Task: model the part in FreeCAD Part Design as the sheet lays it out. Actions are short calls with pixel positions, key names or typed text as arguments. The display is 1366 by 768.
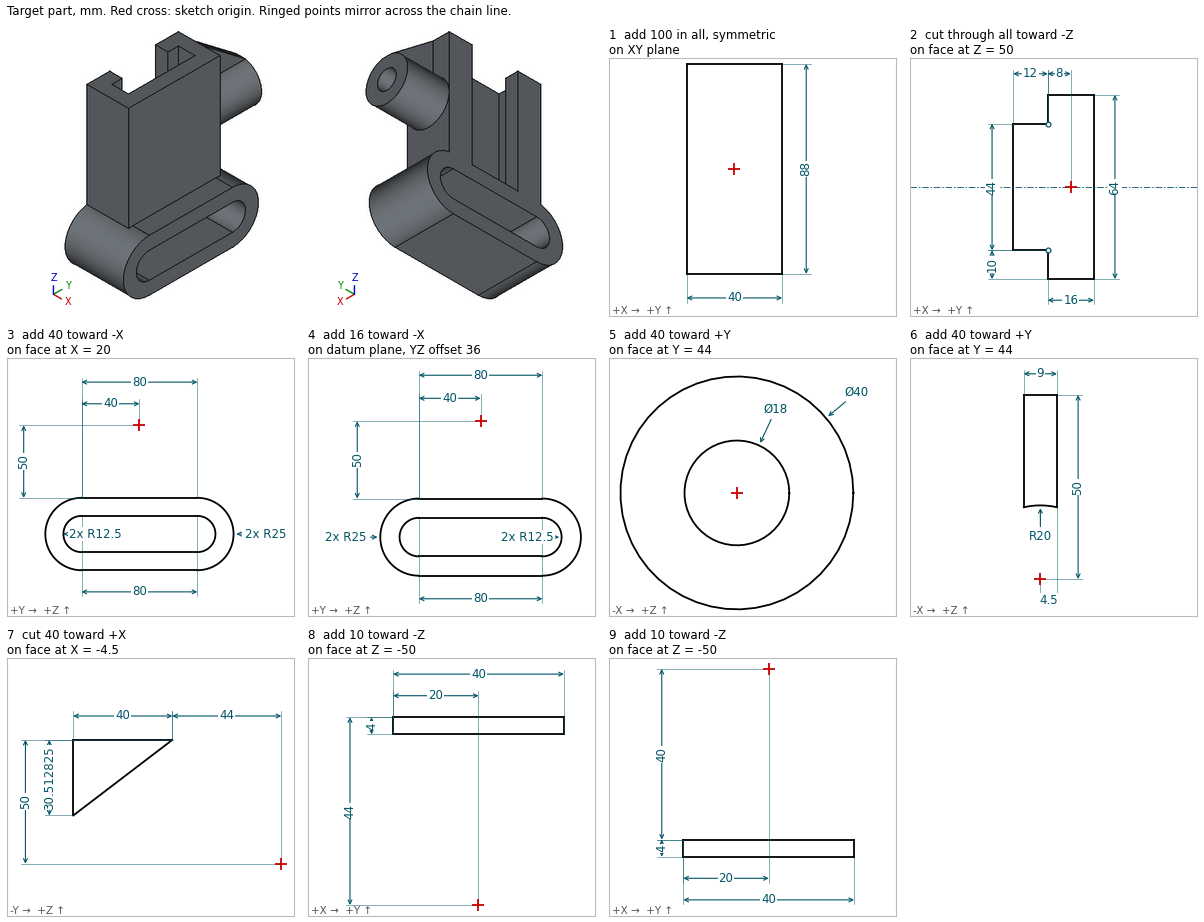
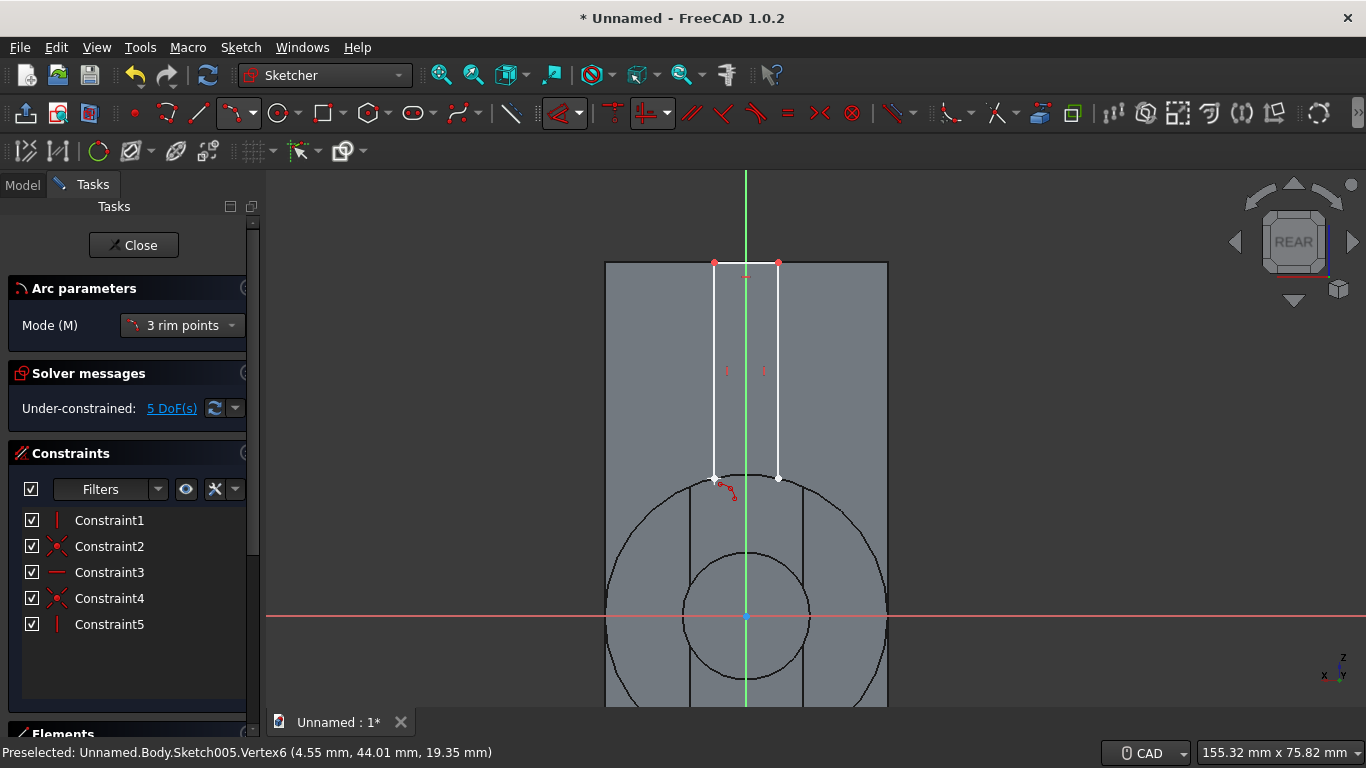
click(714, 479)
click(778, 479)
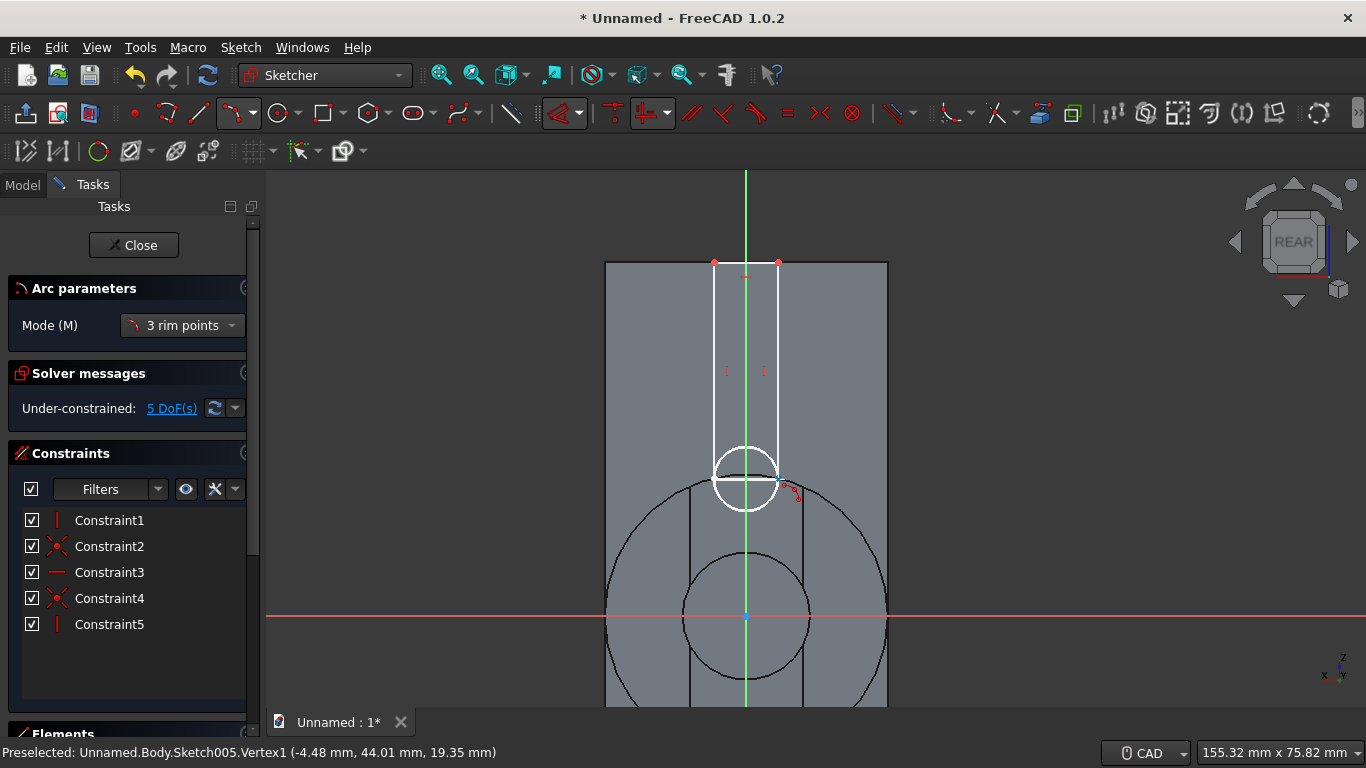
scroll(740, 475, up, 8)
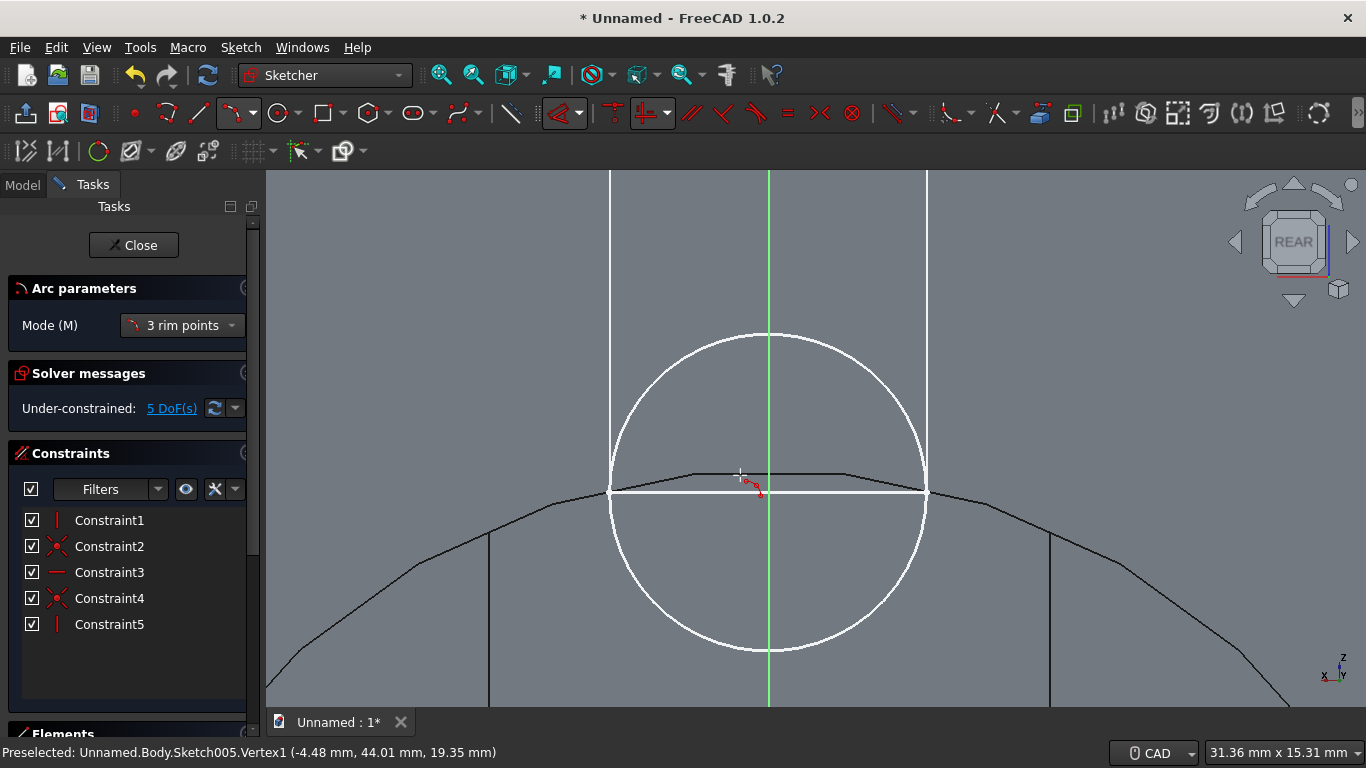
click(737, 471)
key(Escape)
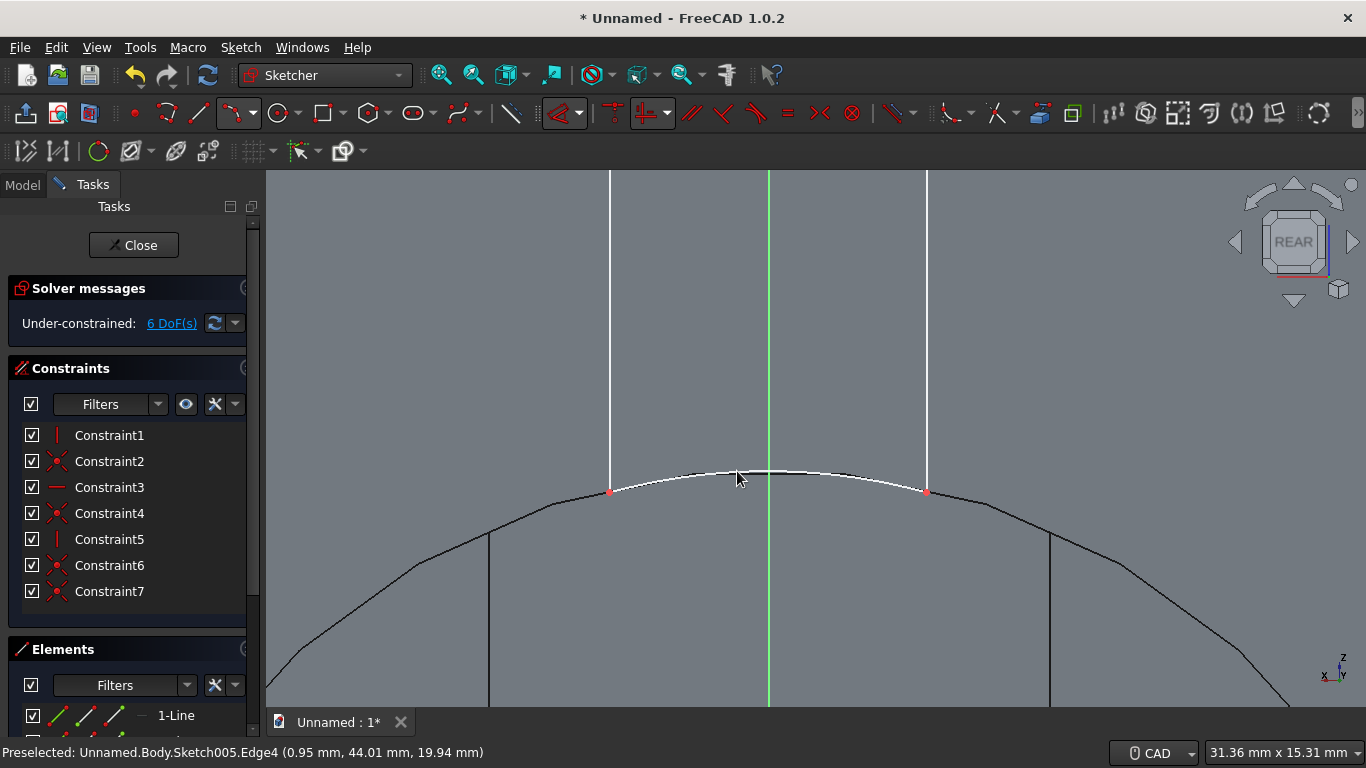
scroll(742, 475, down, 8)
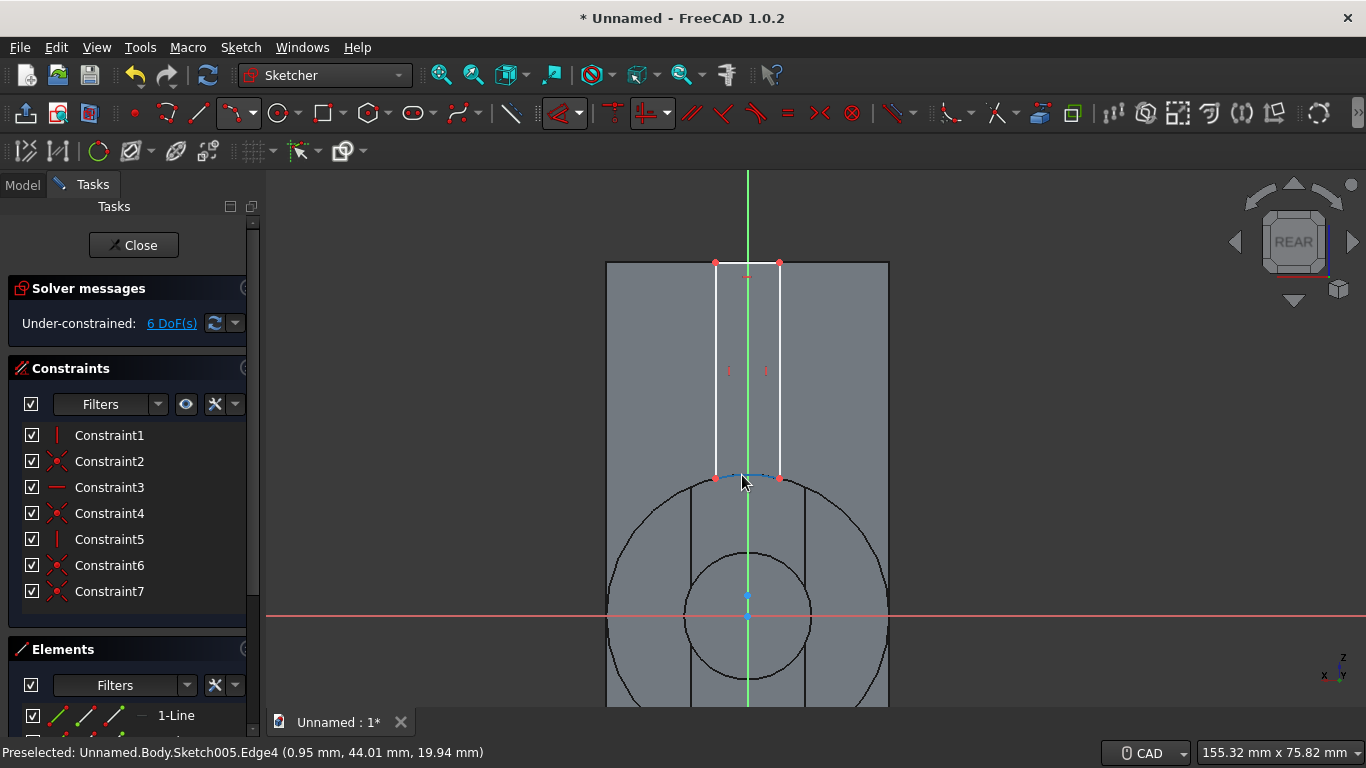
drag(738, 586, 758, 626)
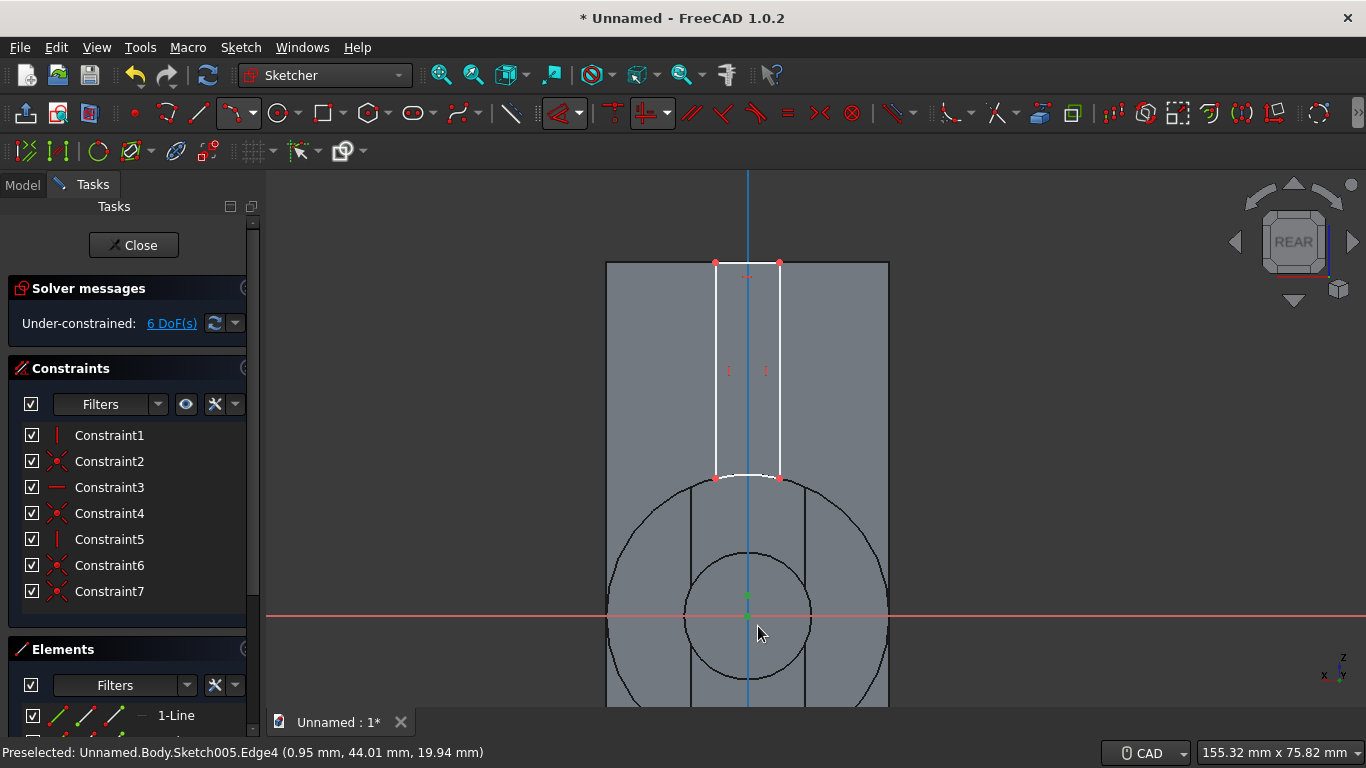
key(c)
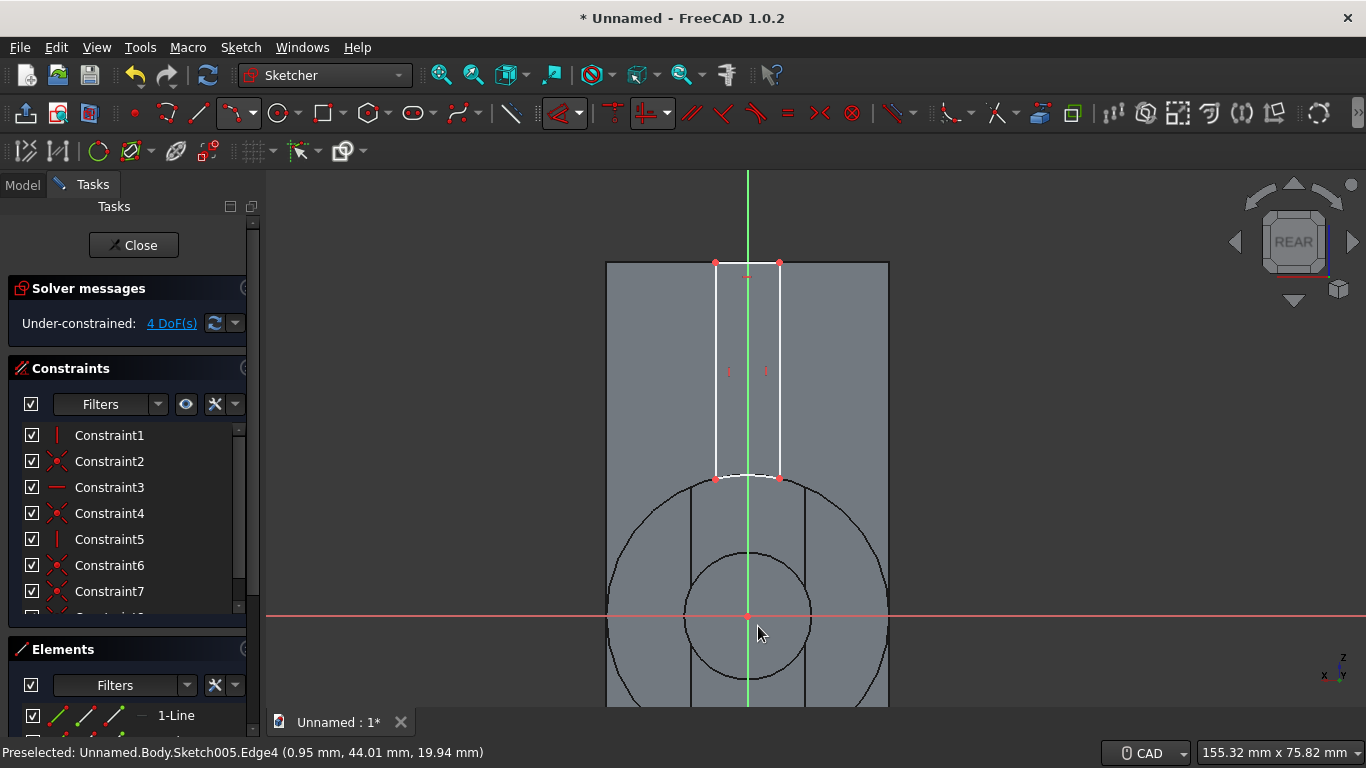
click(760, 476)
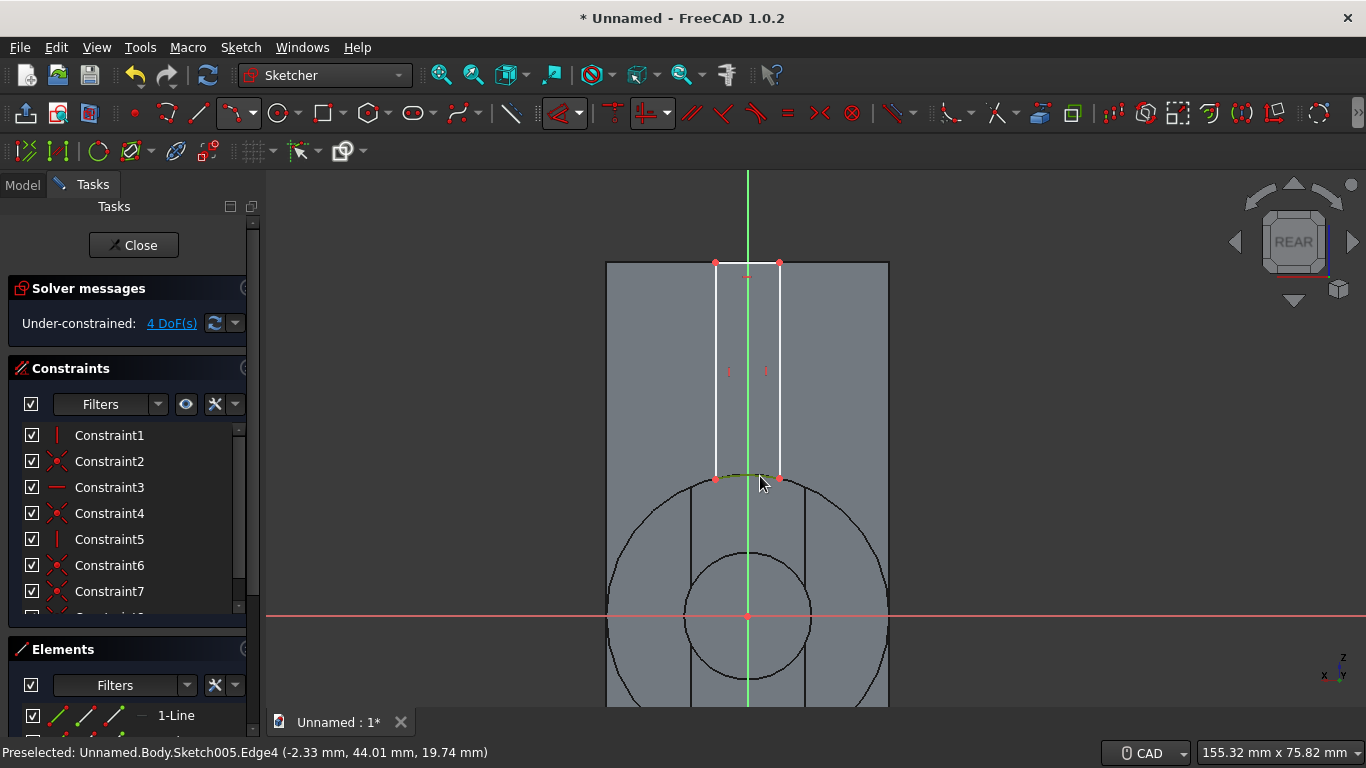
click(582, 114)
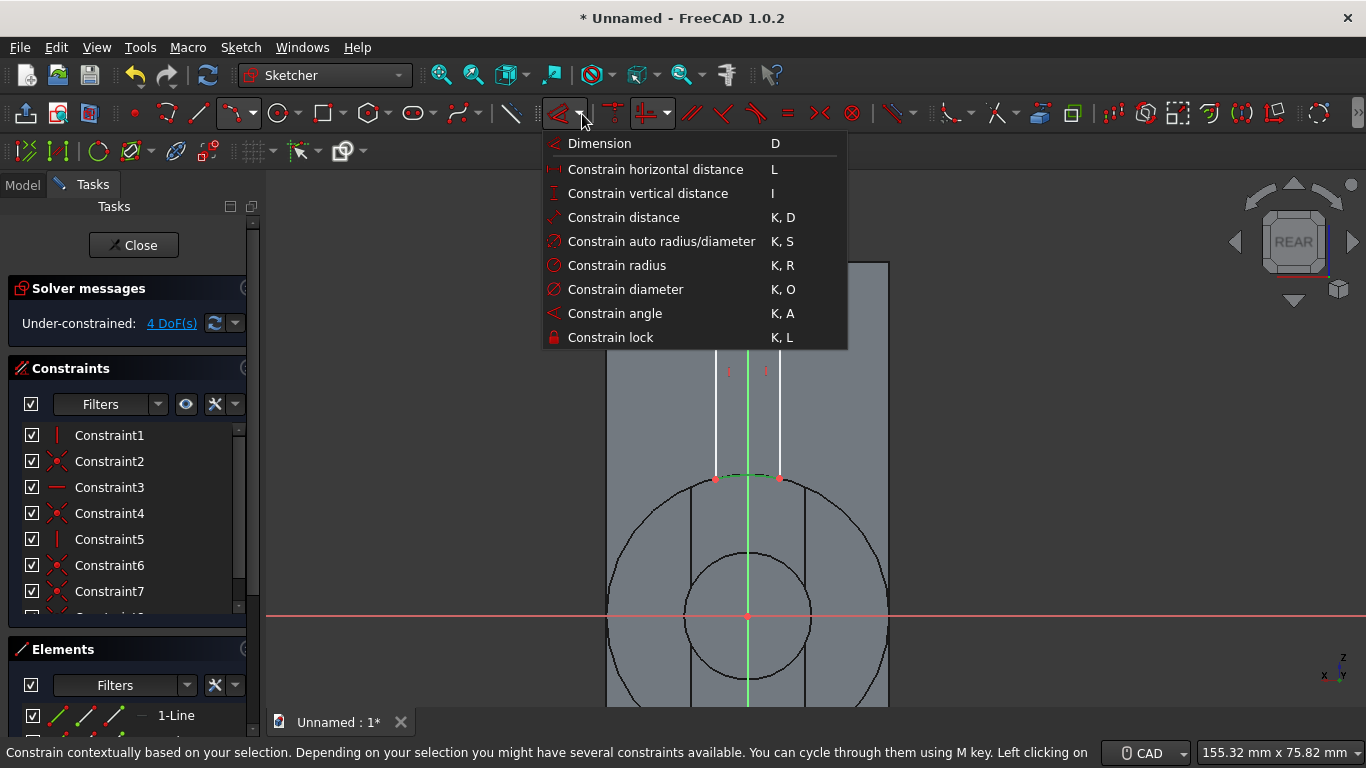
click(695, 265)